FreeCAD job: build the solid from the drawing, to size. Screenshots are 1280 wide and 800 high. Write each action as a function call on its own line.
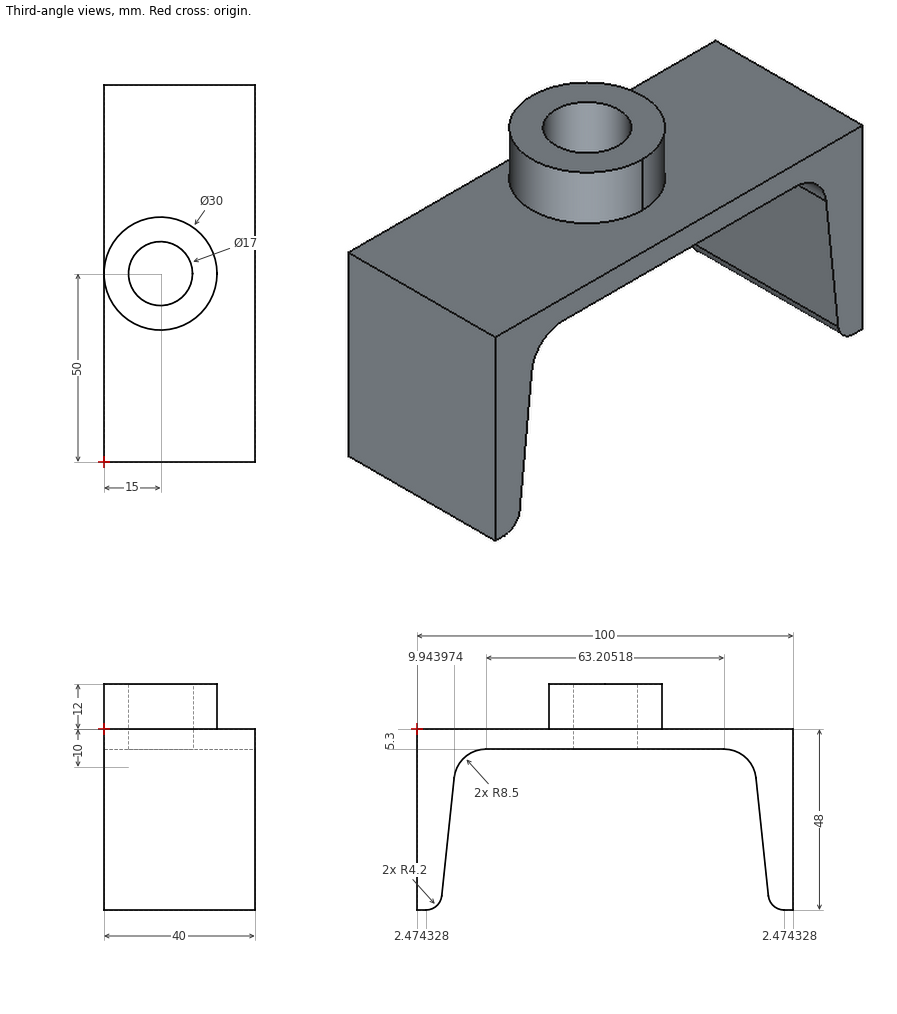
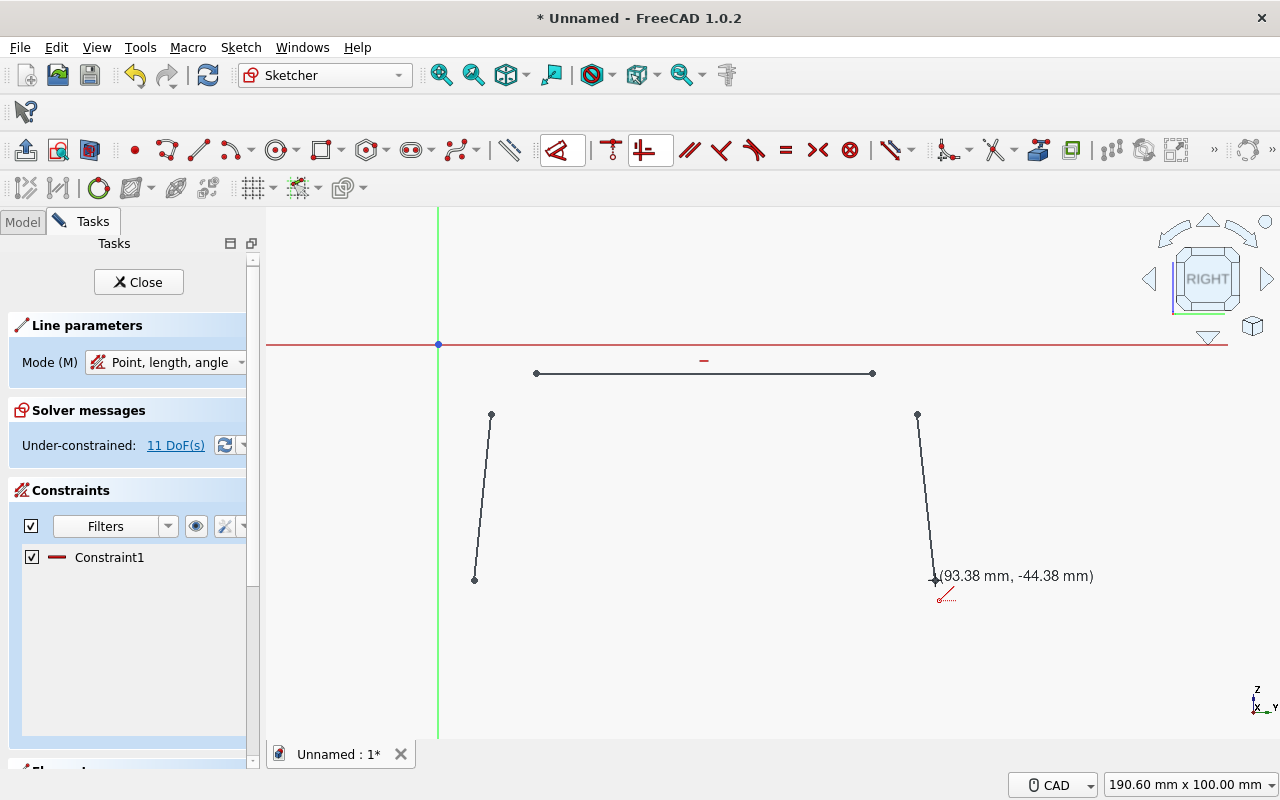
click(168, 150)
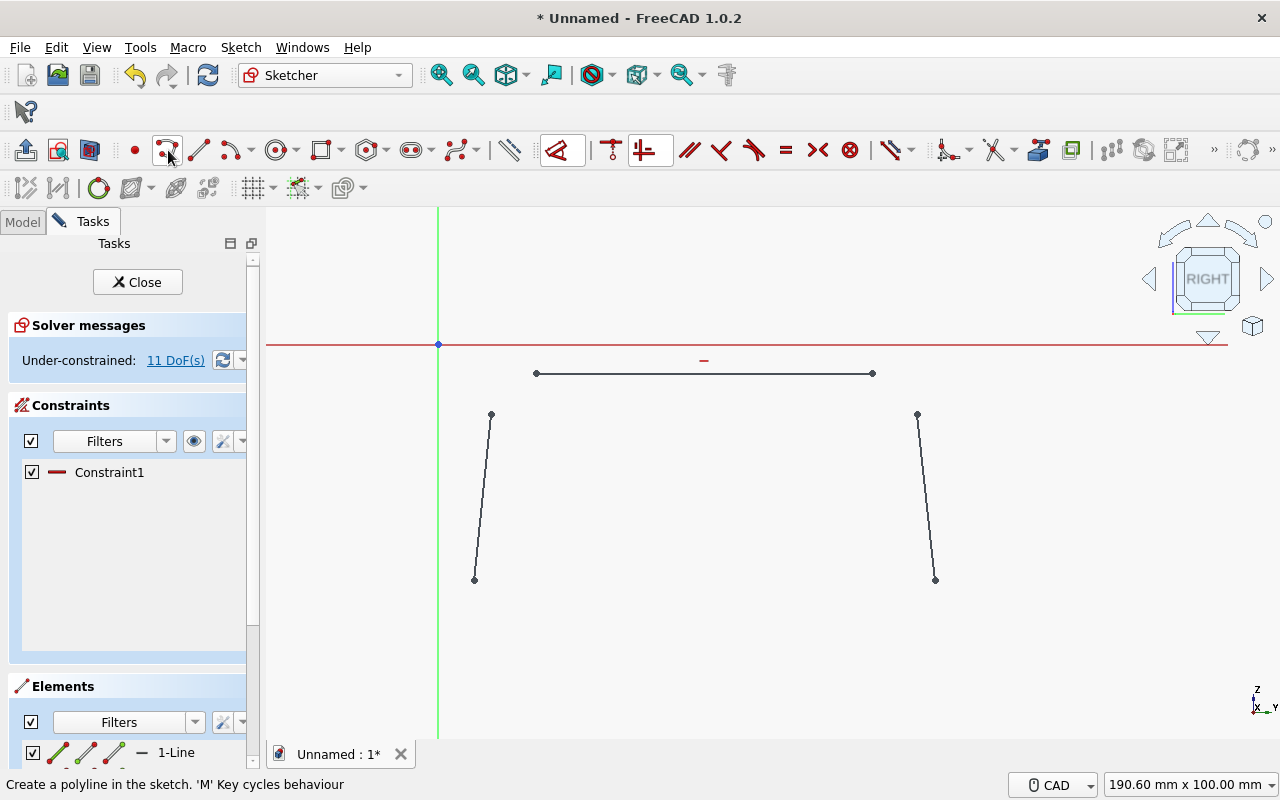
click(957, 600)
click(970, 600)
click(970, 345)
click(438, 345)
click(447, 600)
click(451, 600)
right_click(451, 600)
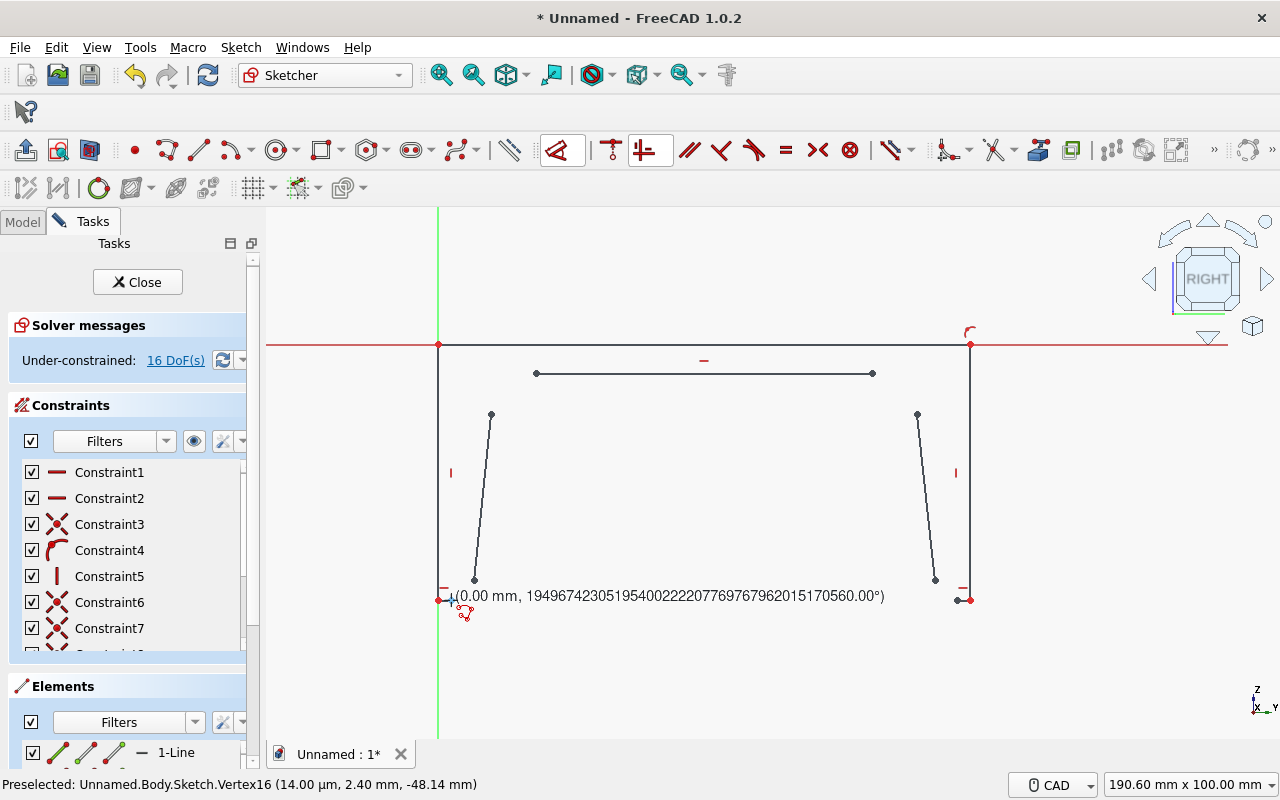
click(254, 150)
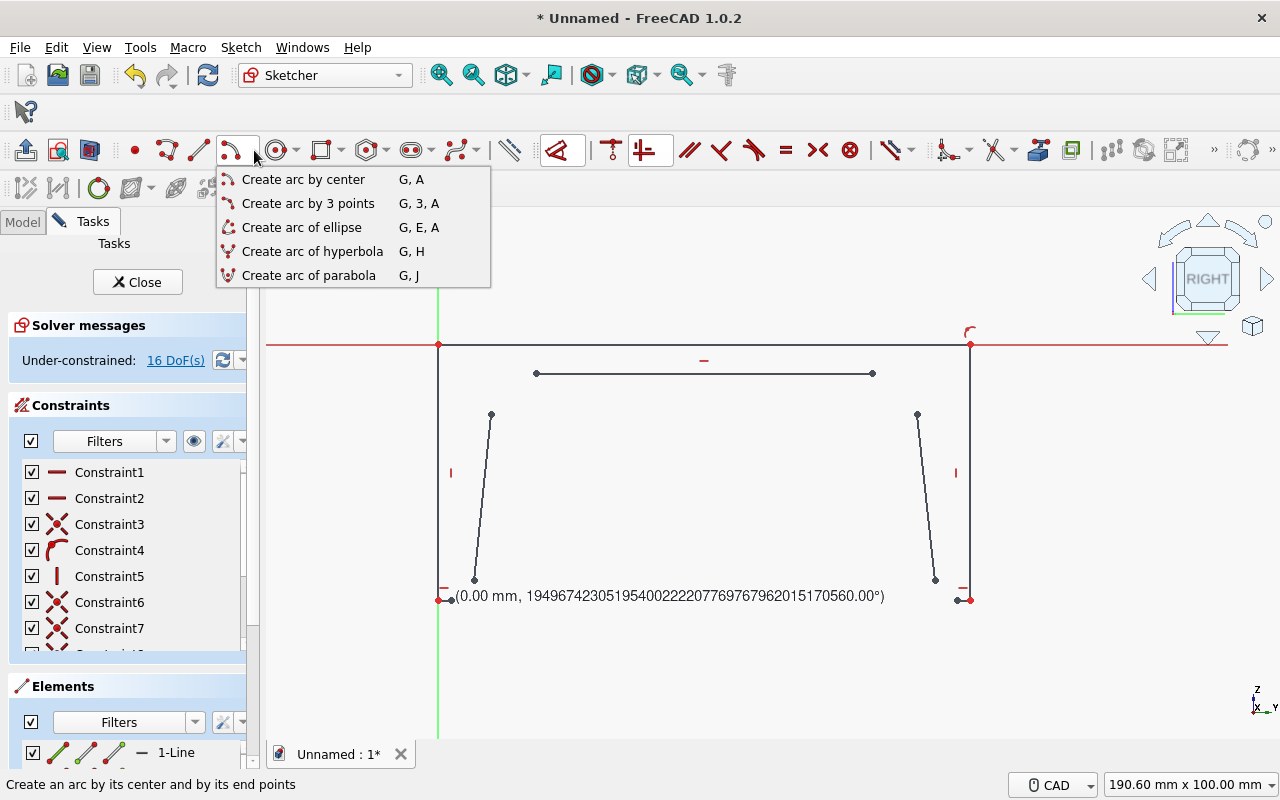
click(354, 203)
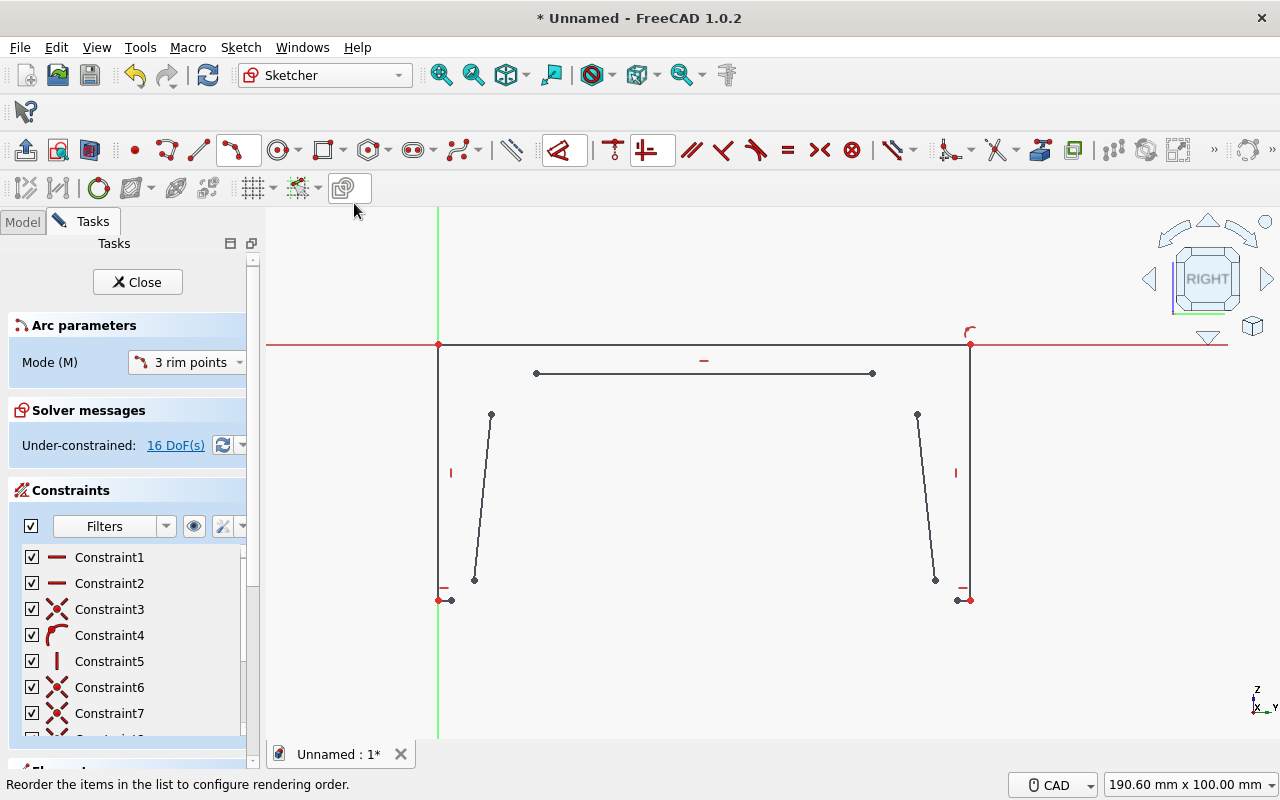
click(491, 415)
click(536, 374)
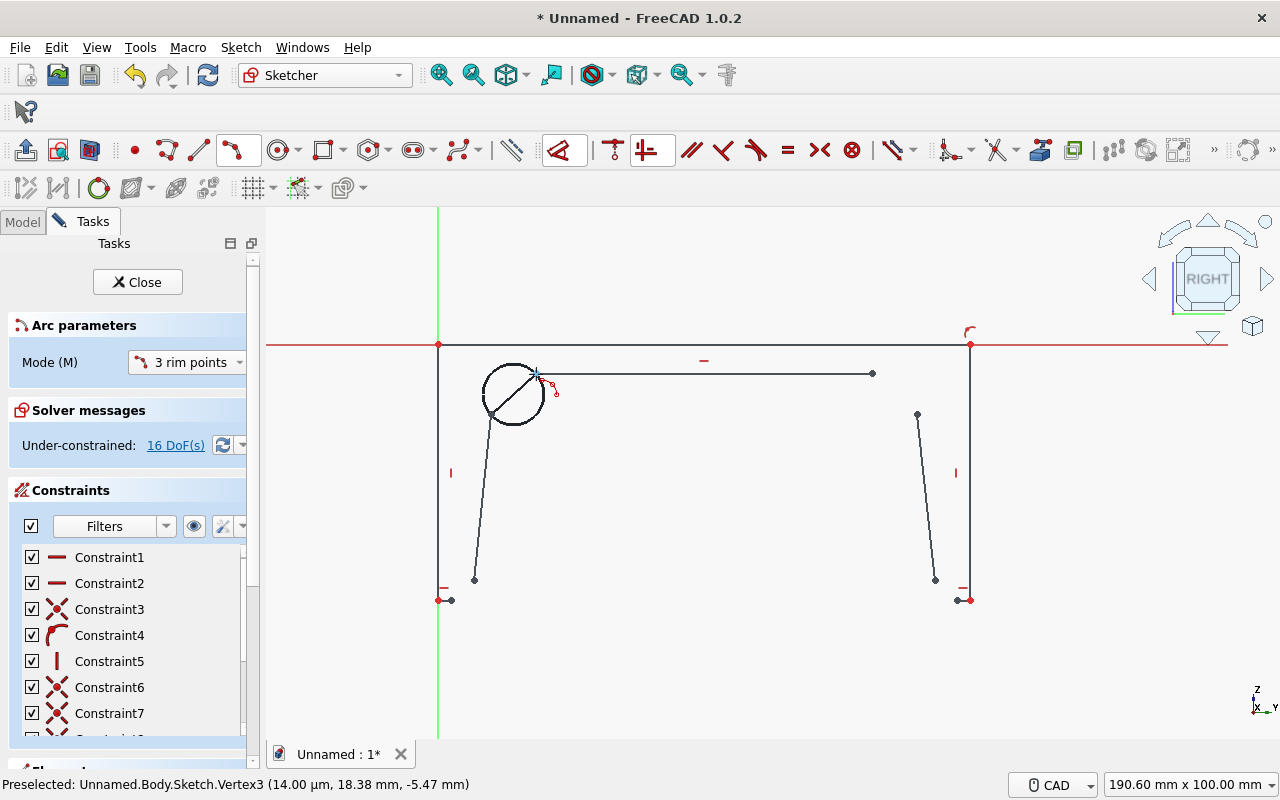
scroll(506, 385, up, 2)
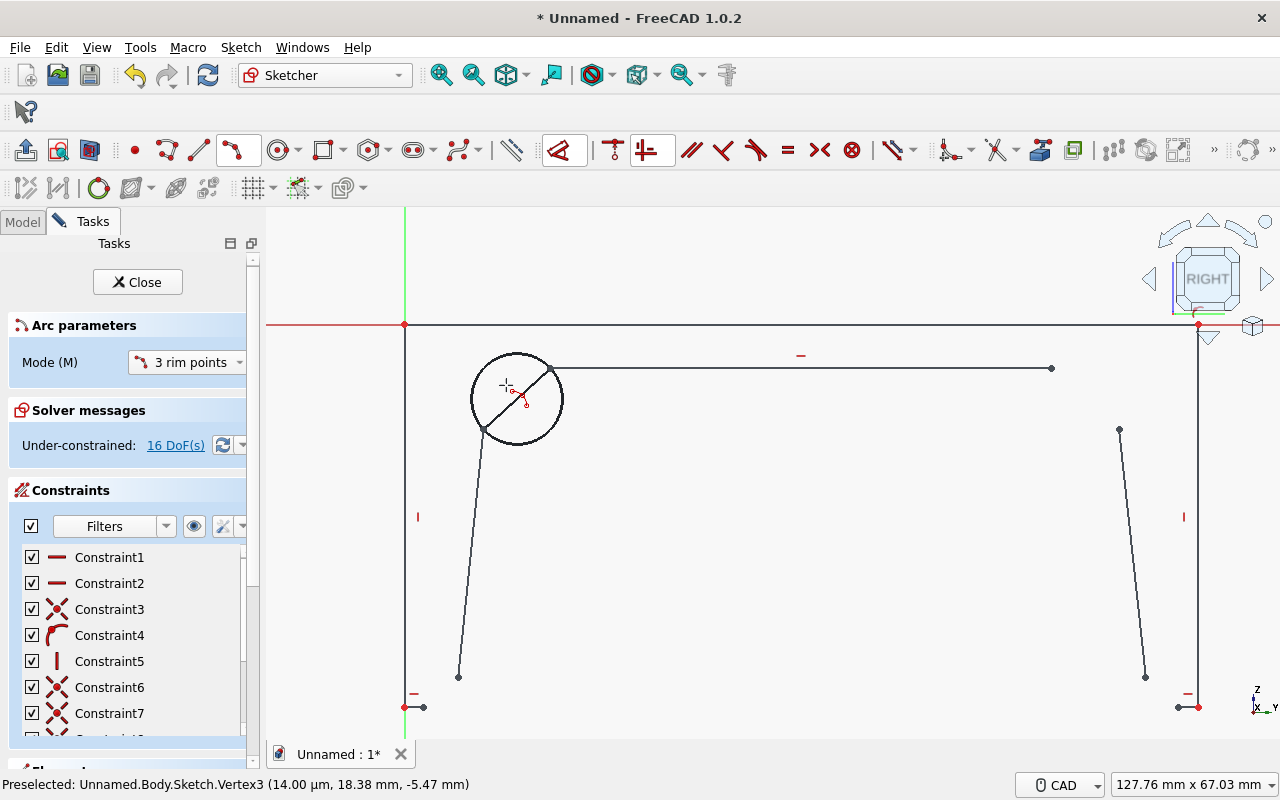
click(506, 384)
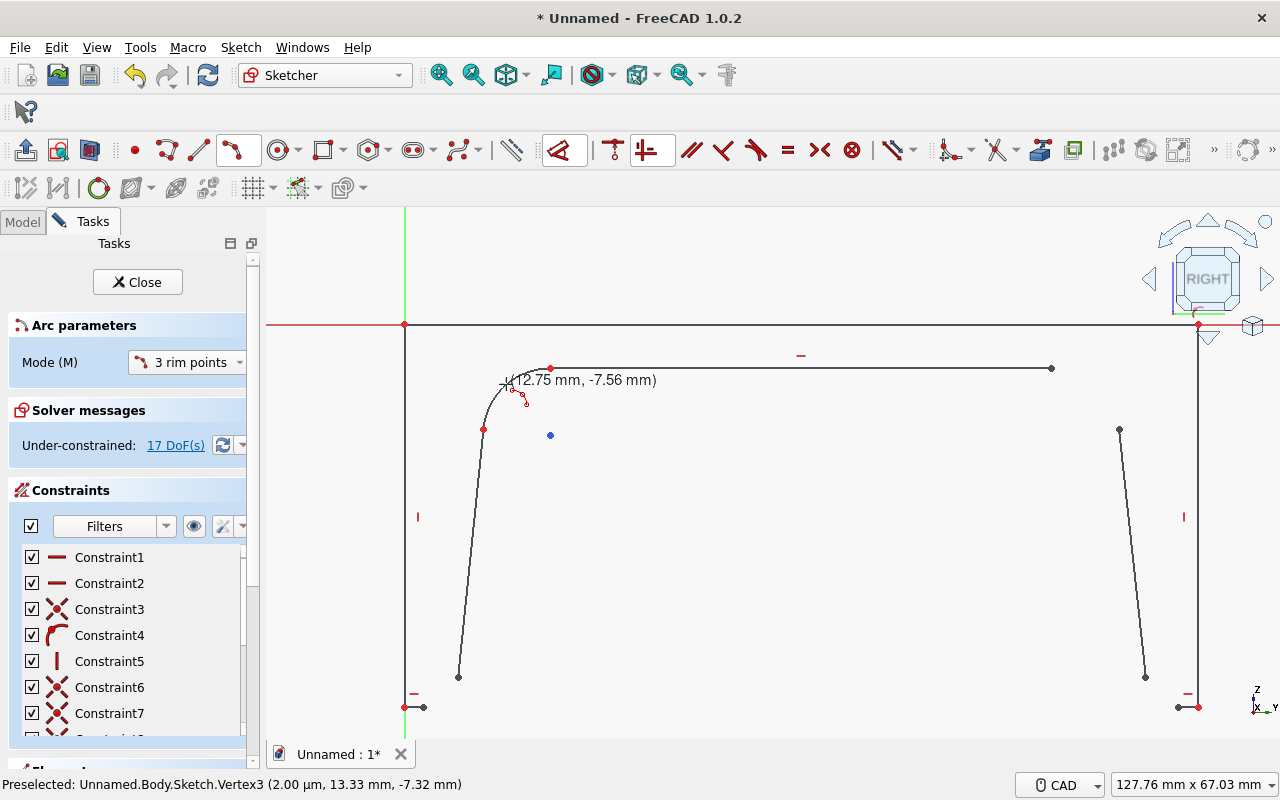
click(1052, 368)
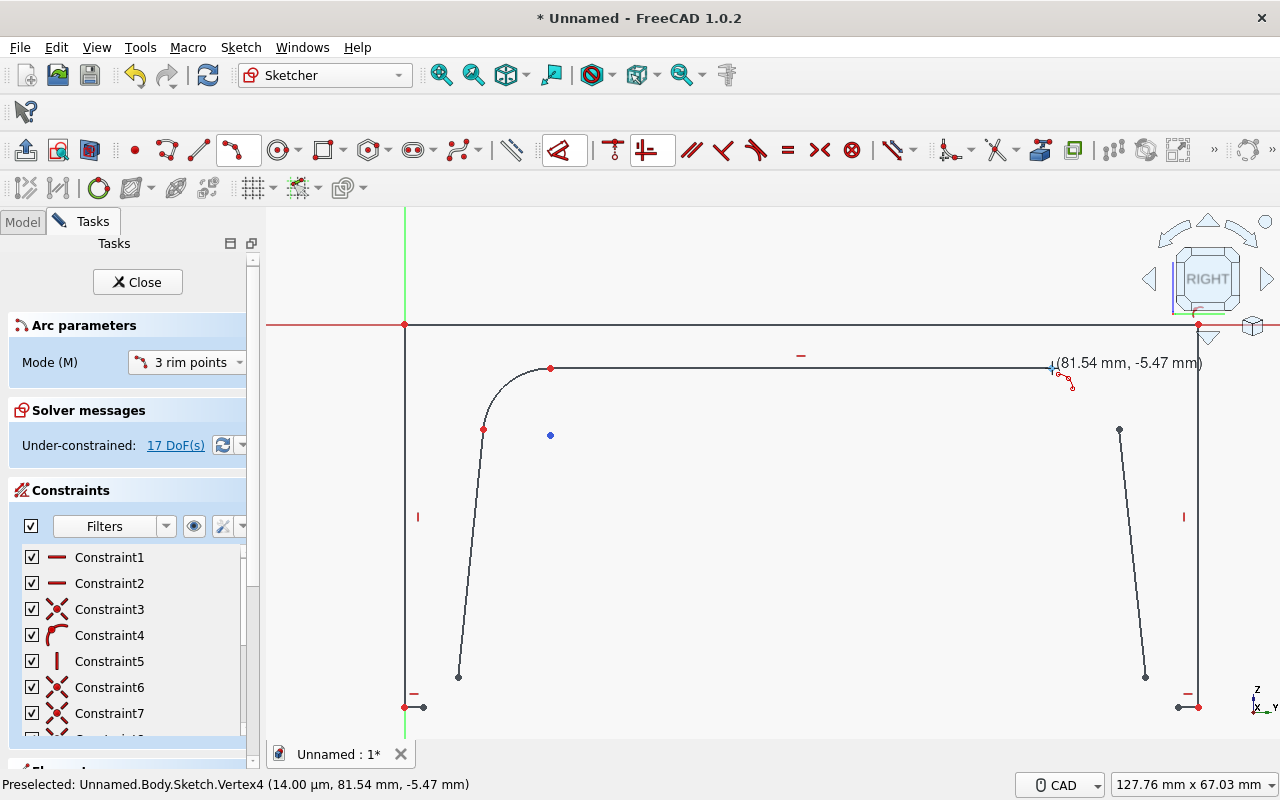
scroll(507, 387, down, 2)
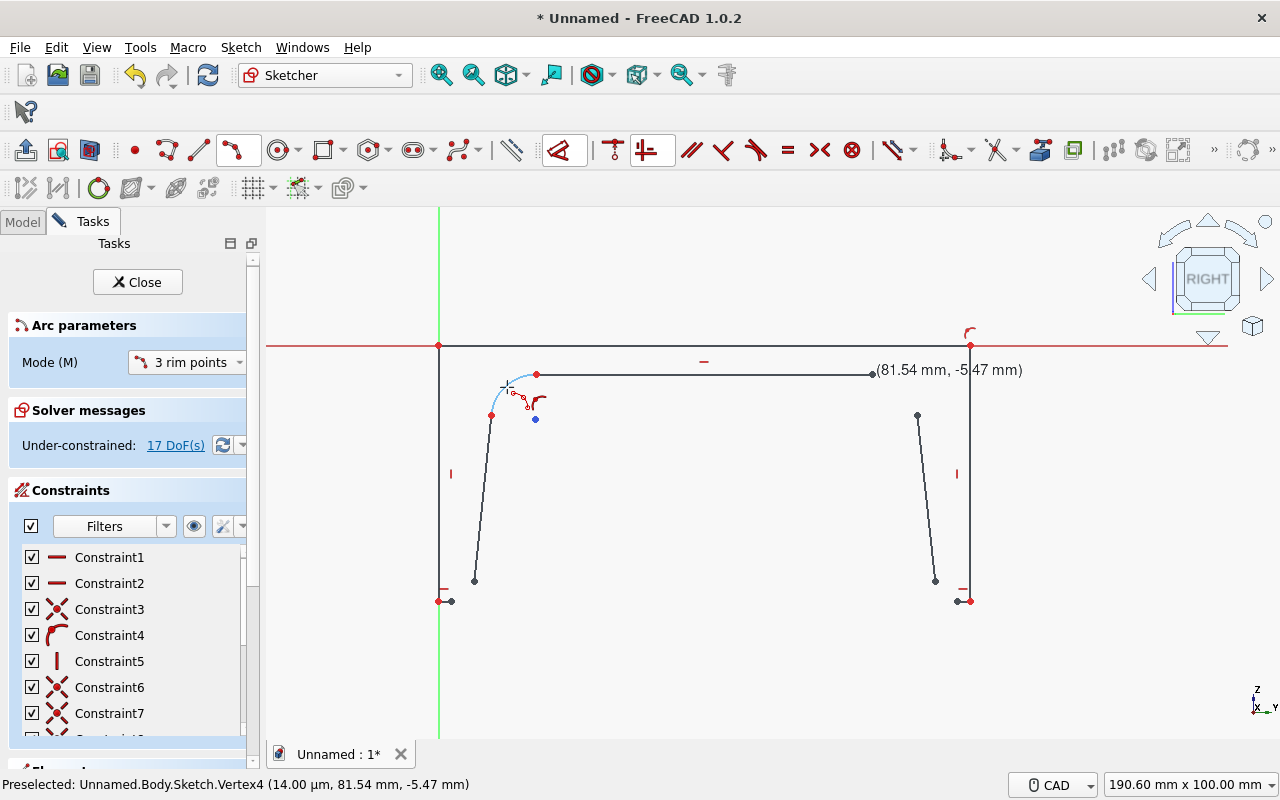
click(917, 416)